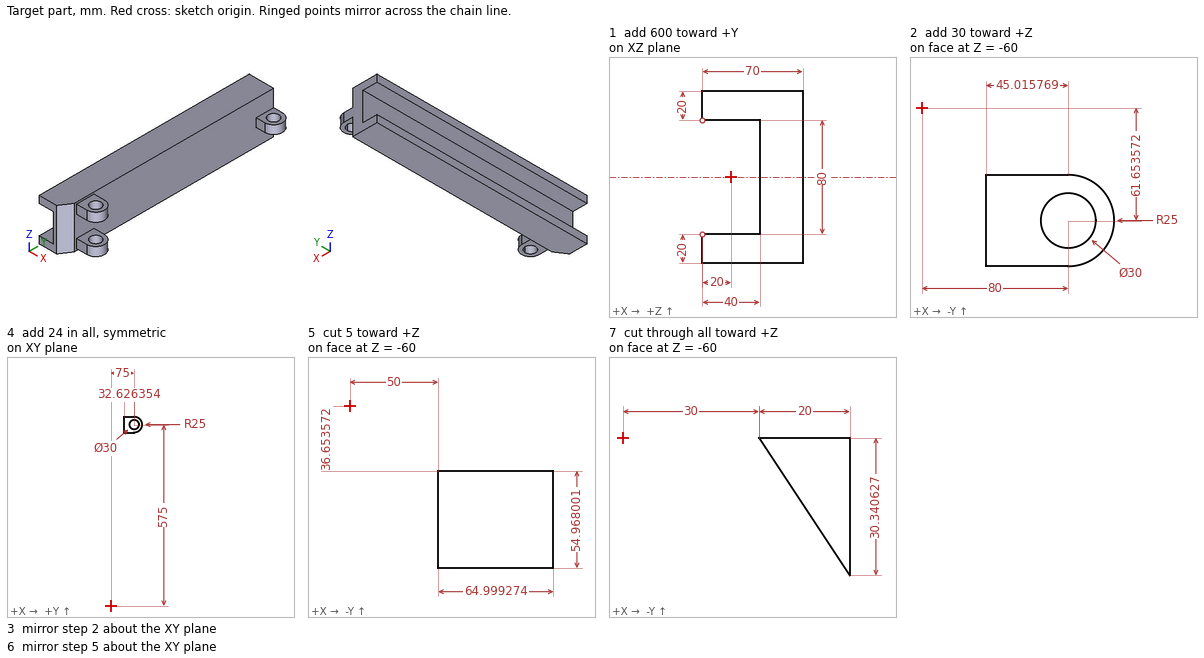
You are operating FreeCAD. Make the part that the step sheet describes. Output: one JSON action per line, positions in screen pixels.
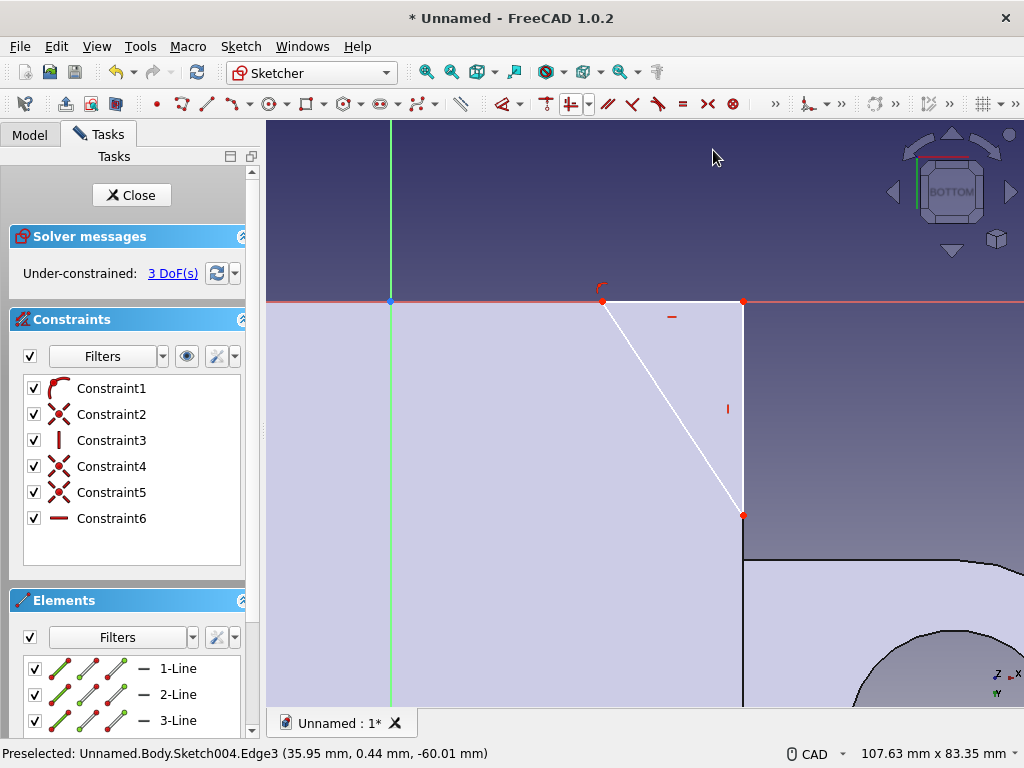
{"action": "left_click", "coordinate": [502, 104]}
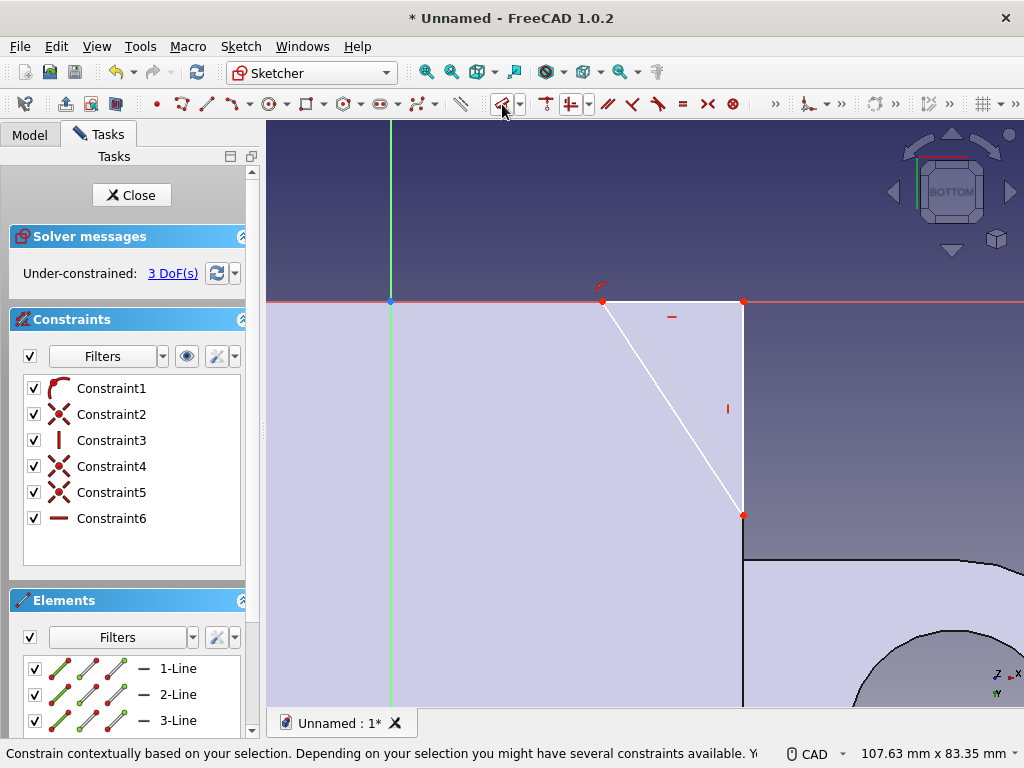
{"action": "left_click", "coordinate": [701, 302]}
{"action": "left_click", "coordinate": [672, 268]}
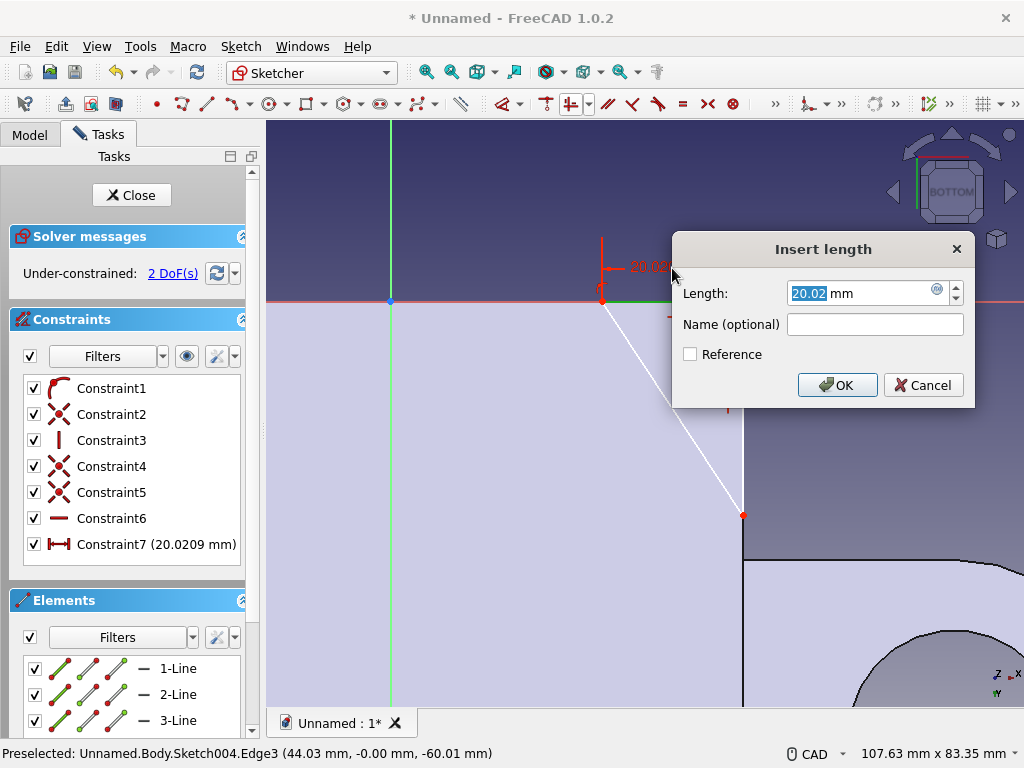
{"action": "type", "text": "20"}
{"action": "key", "text": "Return"}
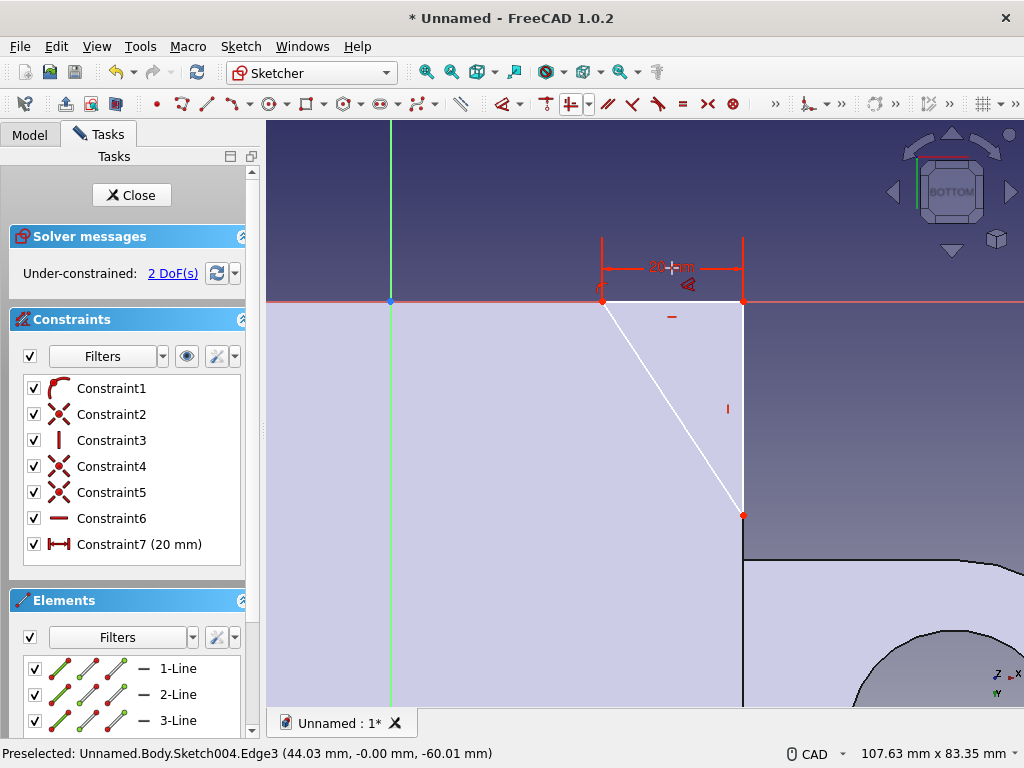
{"action": "left_click", "coordinate": [602, 302]}
{"action": "left_click", "coordinate": [497, 268]}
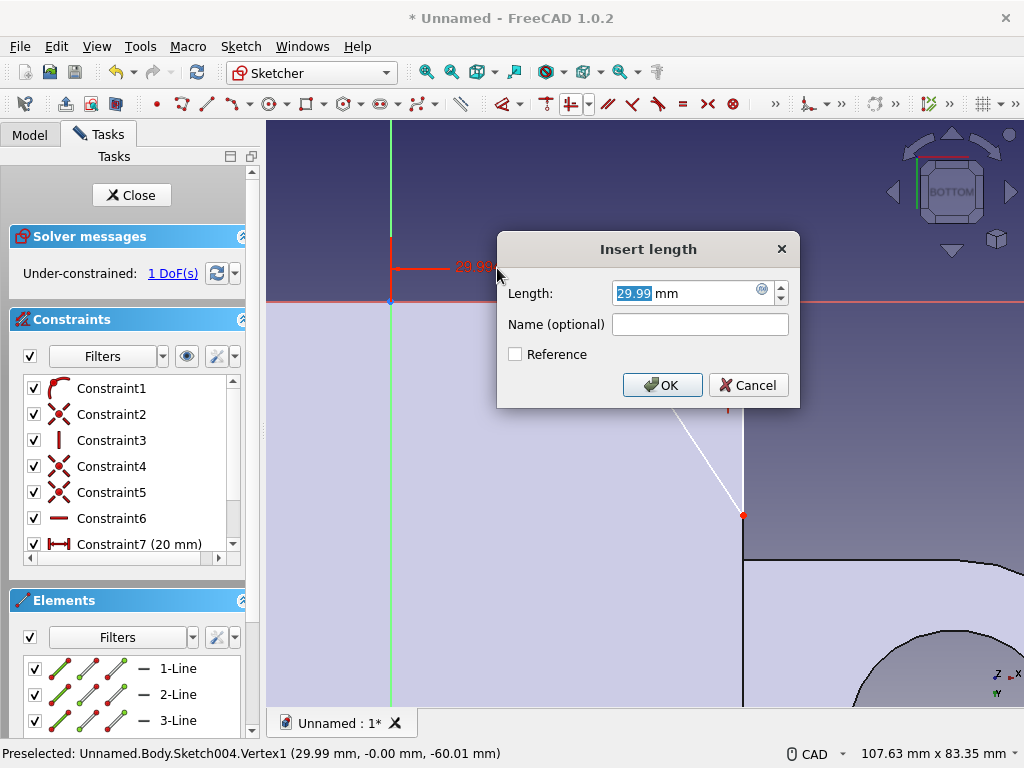
{"action": "type", "text": "30"}
{"action": "key", "text": "Return"}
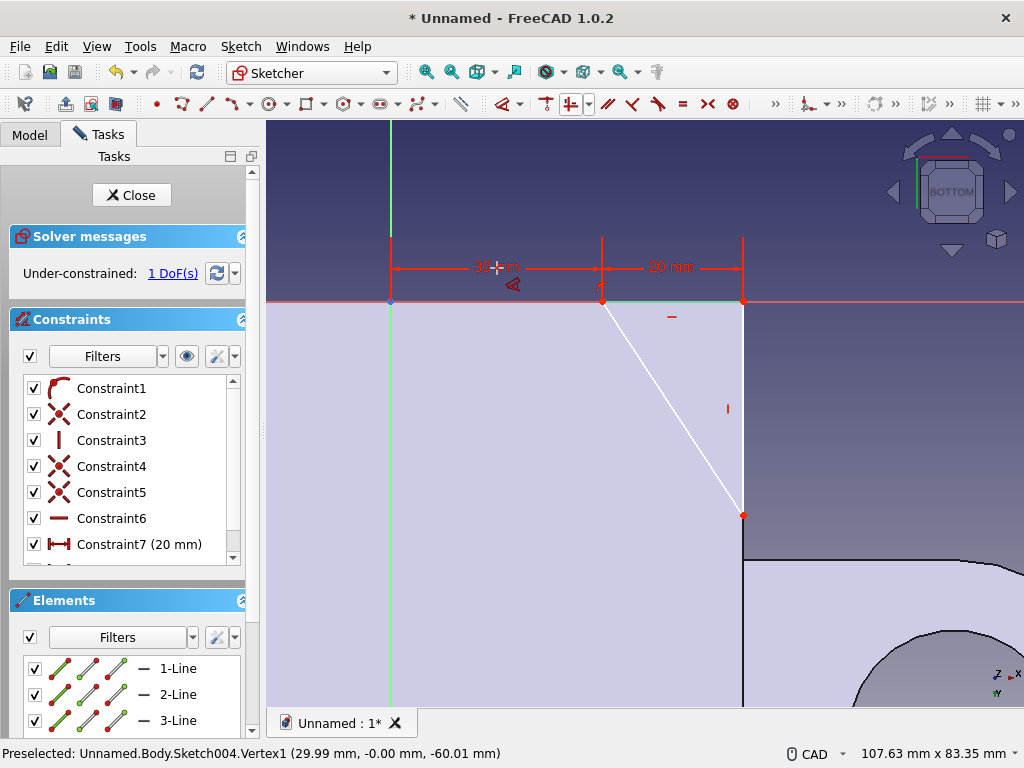
{"action": "left_click", "coordinate": [743, 452]}
{"action": "left_click", "coordinate": [777, 409]}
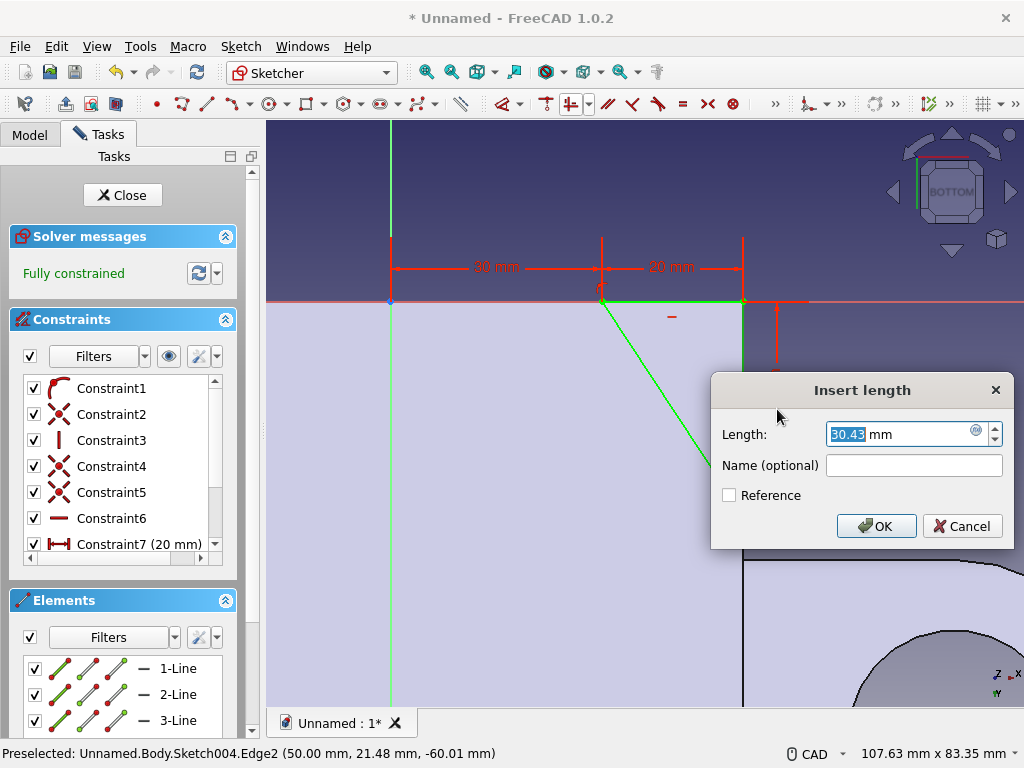
{"action": "type", "text": "30.340627"}
{"action": "key", "text": "Return"}
{"action": "key", "text": "Escape"}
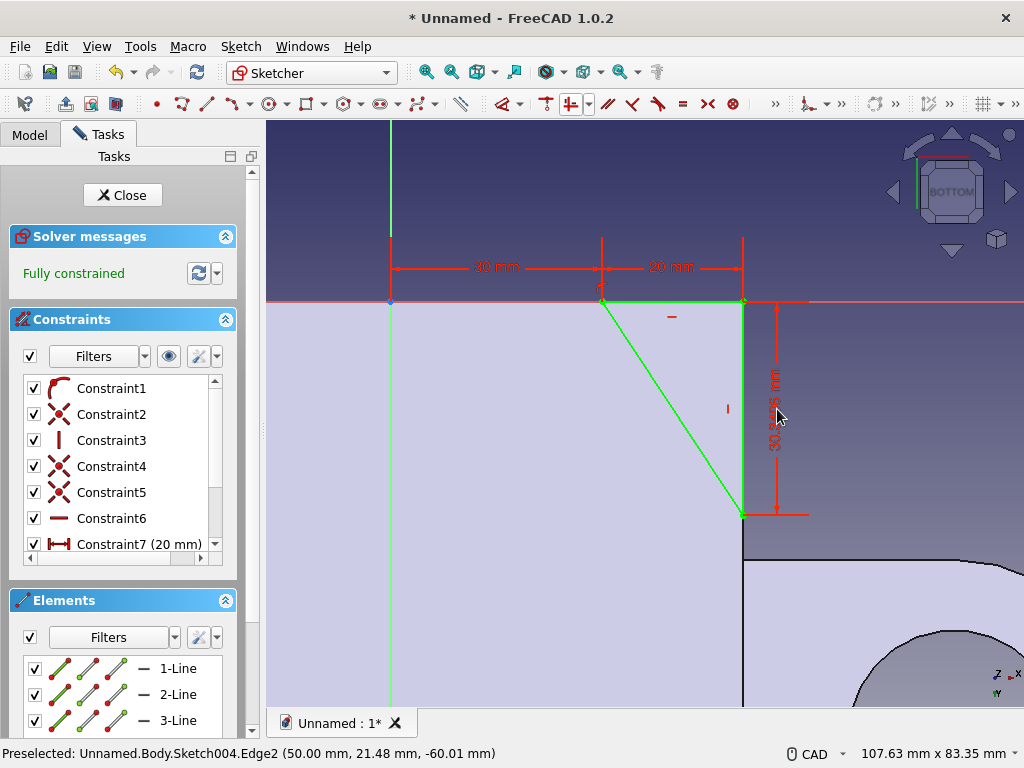
{"action": "left_click", "coordinate": [123, 195]}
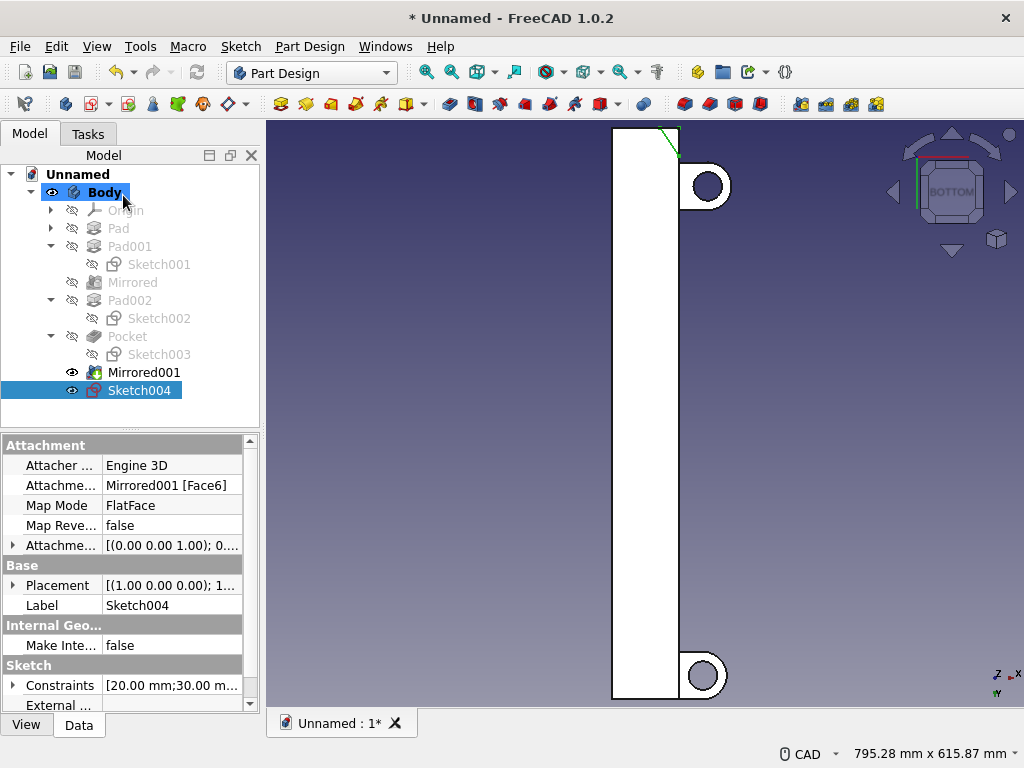
{"action": "left_click", "coordinate": [450, 104]}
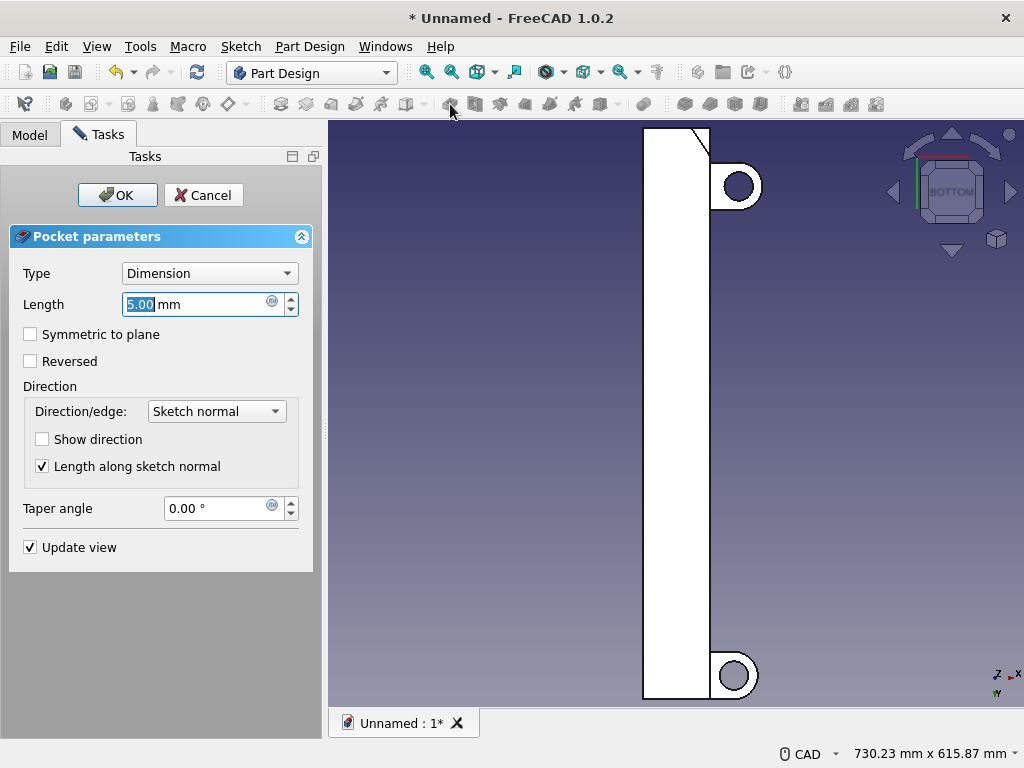
{"action": "left_click", "coordinate": [210, 274]}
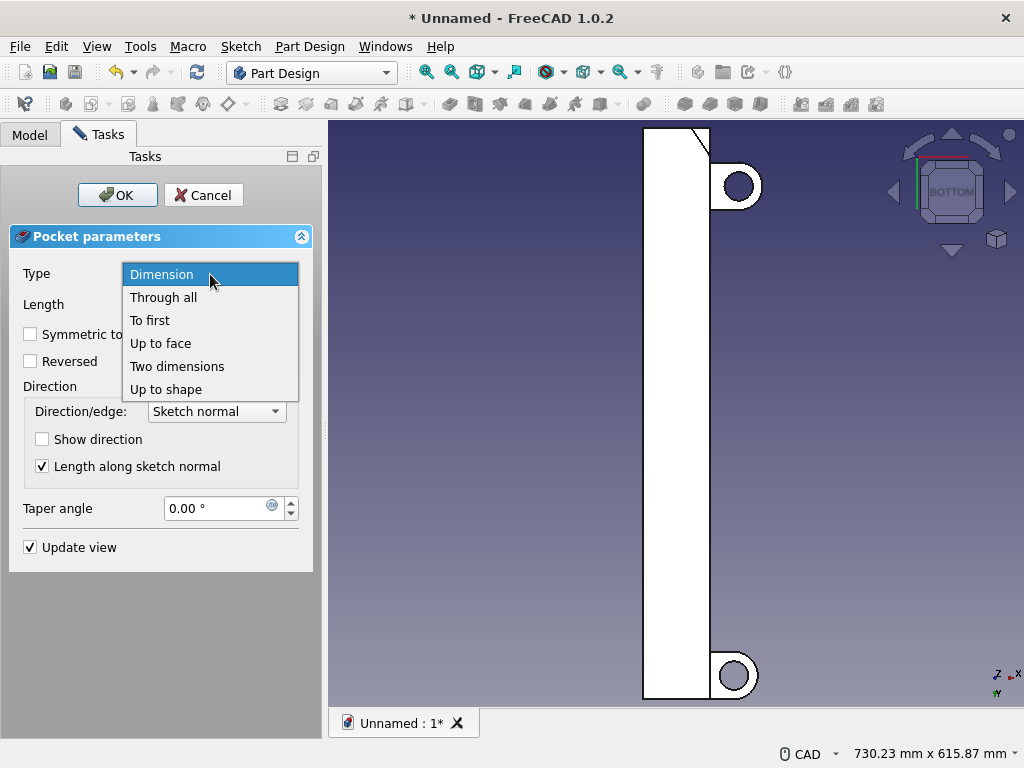
{"action": "left_click", "coordinate": [208, 298]}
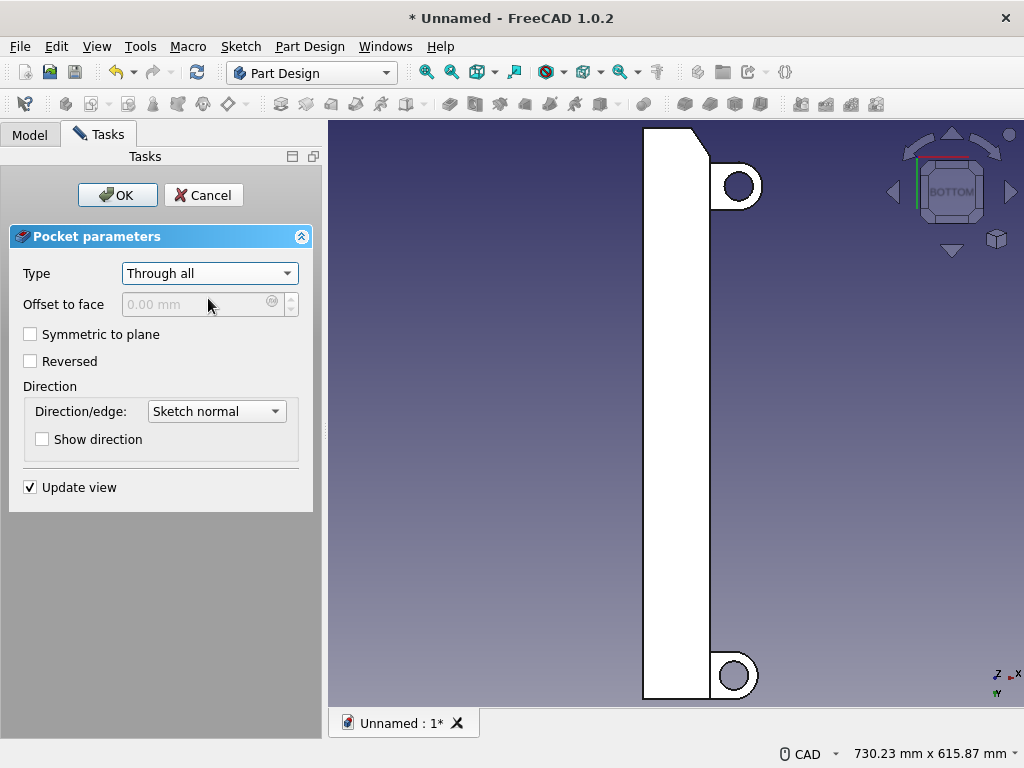
{"action": "left_click", "coordinate": [118, 195]}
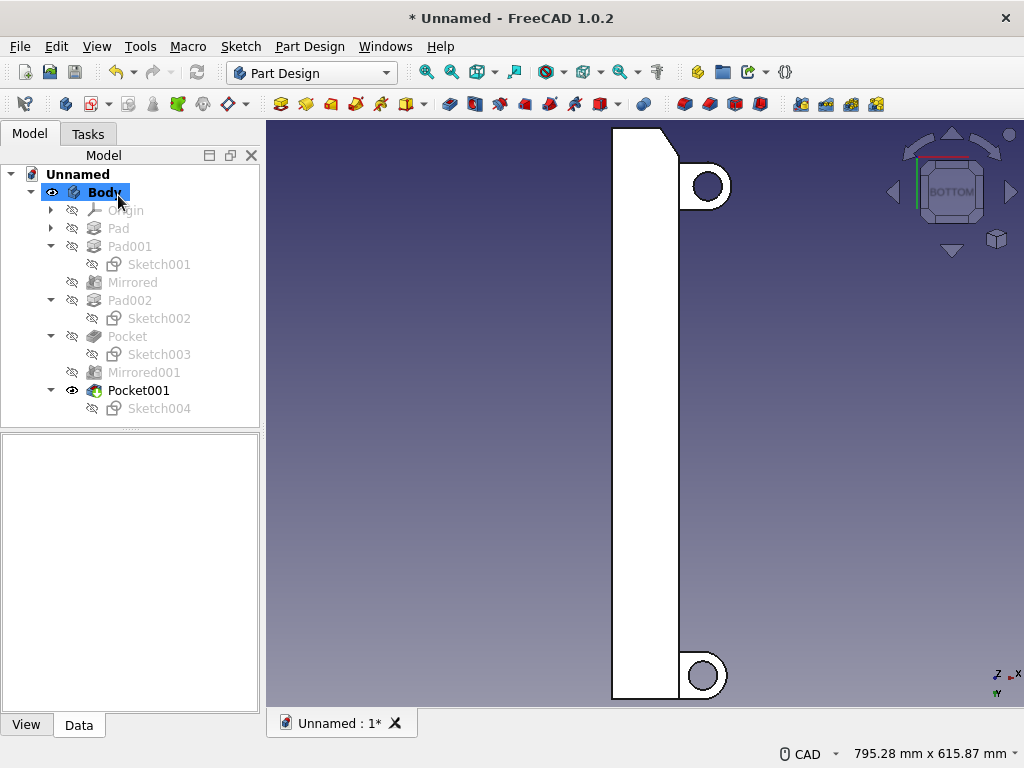
{"action": "key", "text": "0"}